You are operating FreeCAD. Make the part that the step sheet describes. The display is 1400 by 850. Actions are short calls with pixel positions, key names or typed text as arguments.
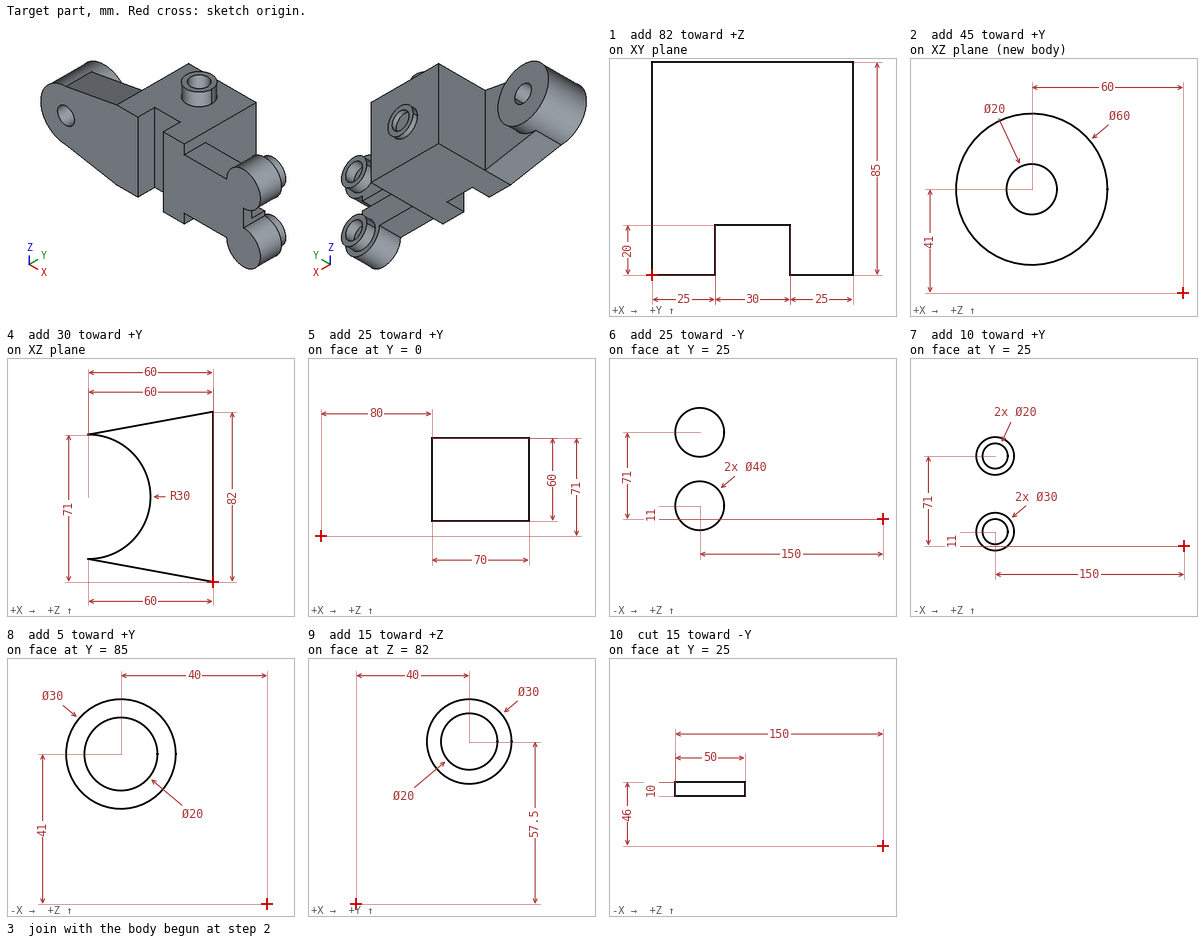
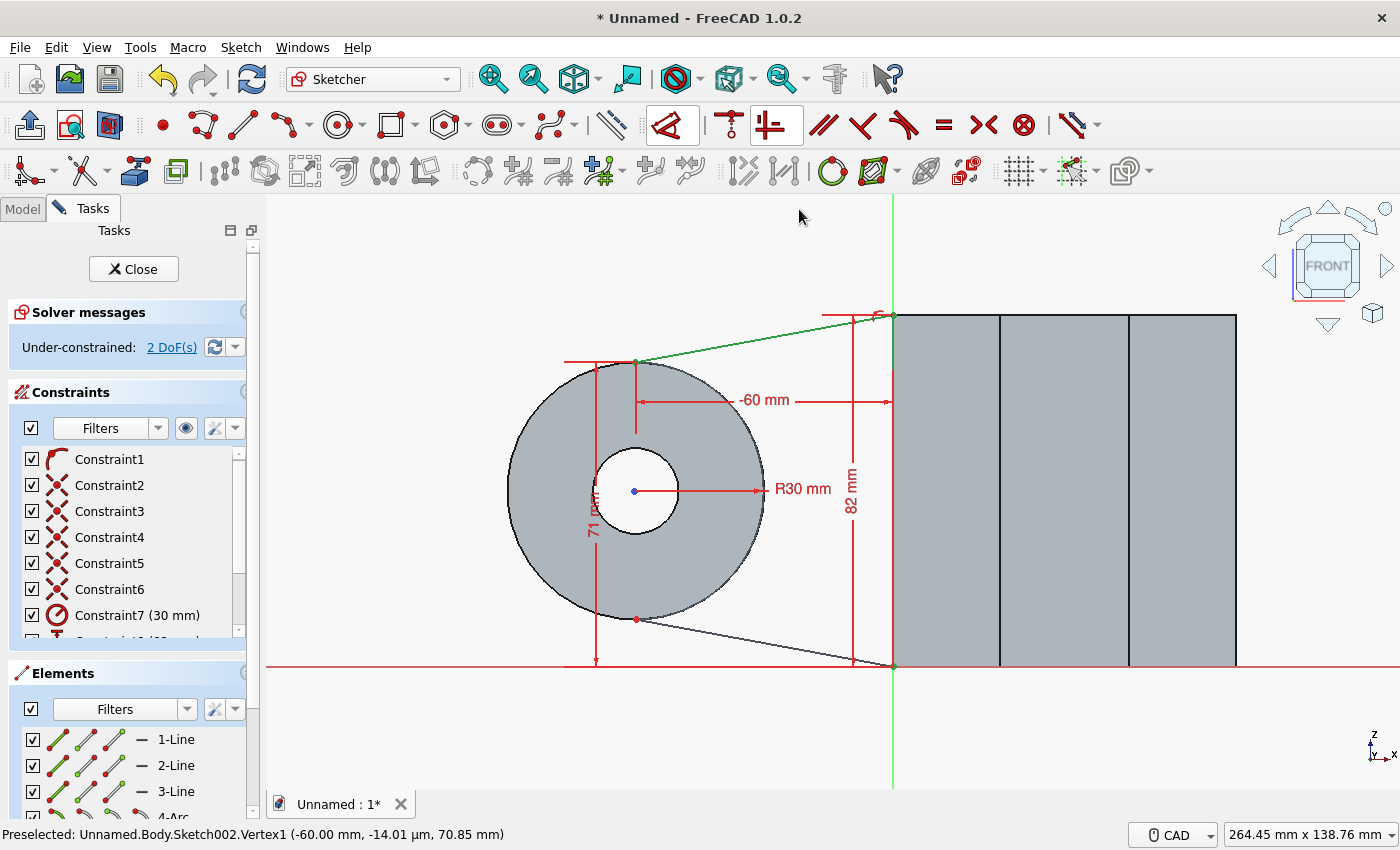
click(636, 620)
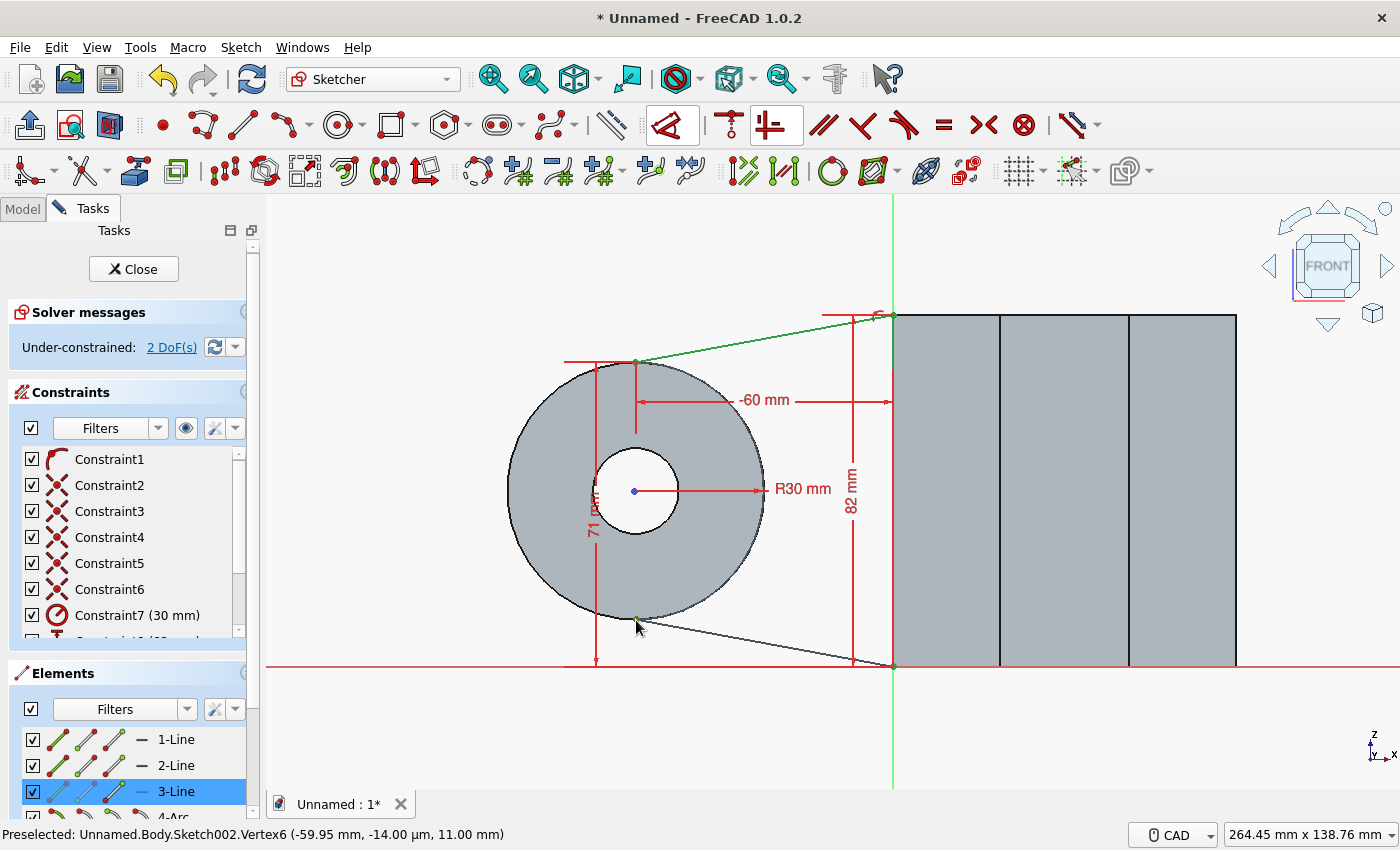
click(694, 126)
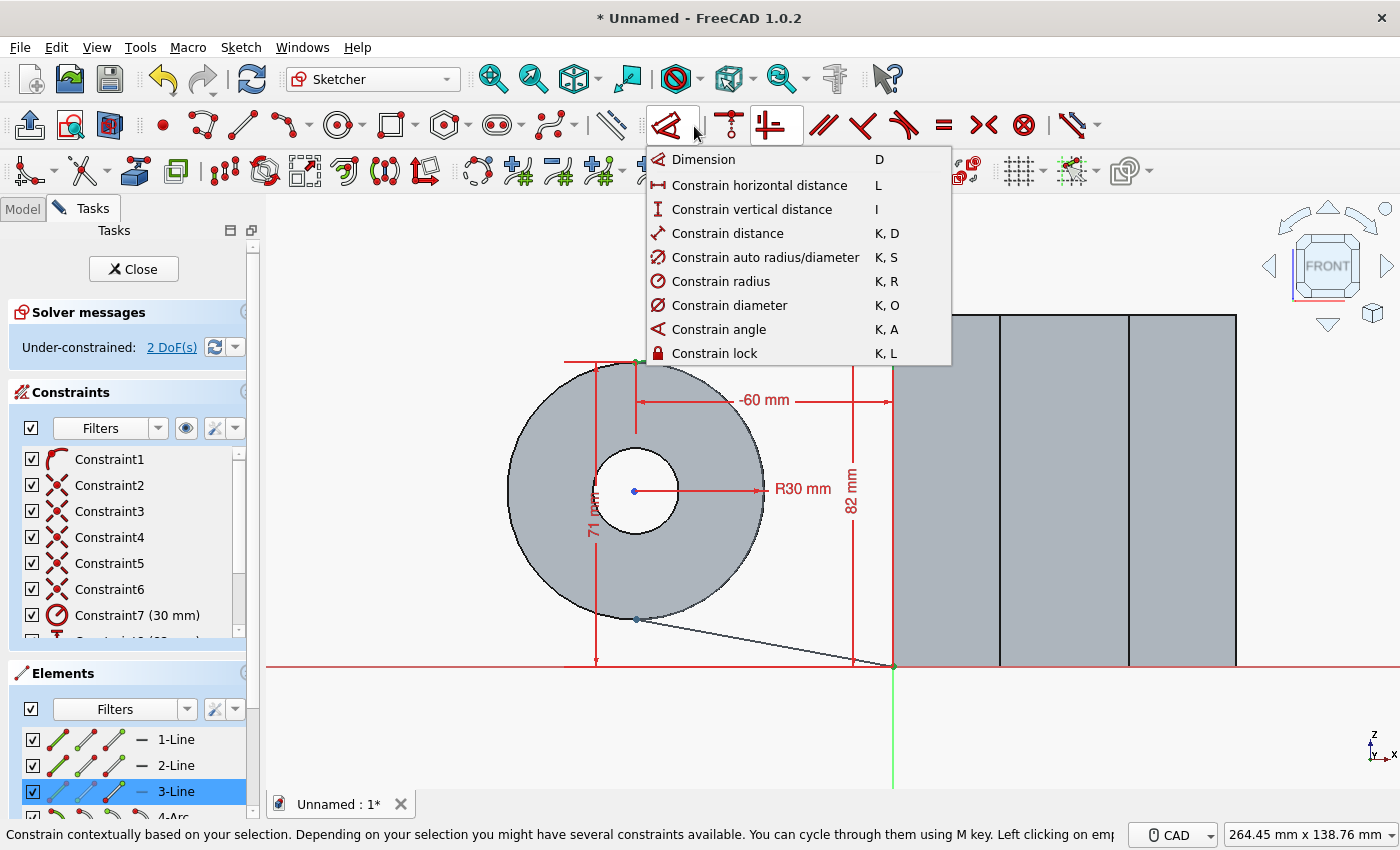
click(799, 185)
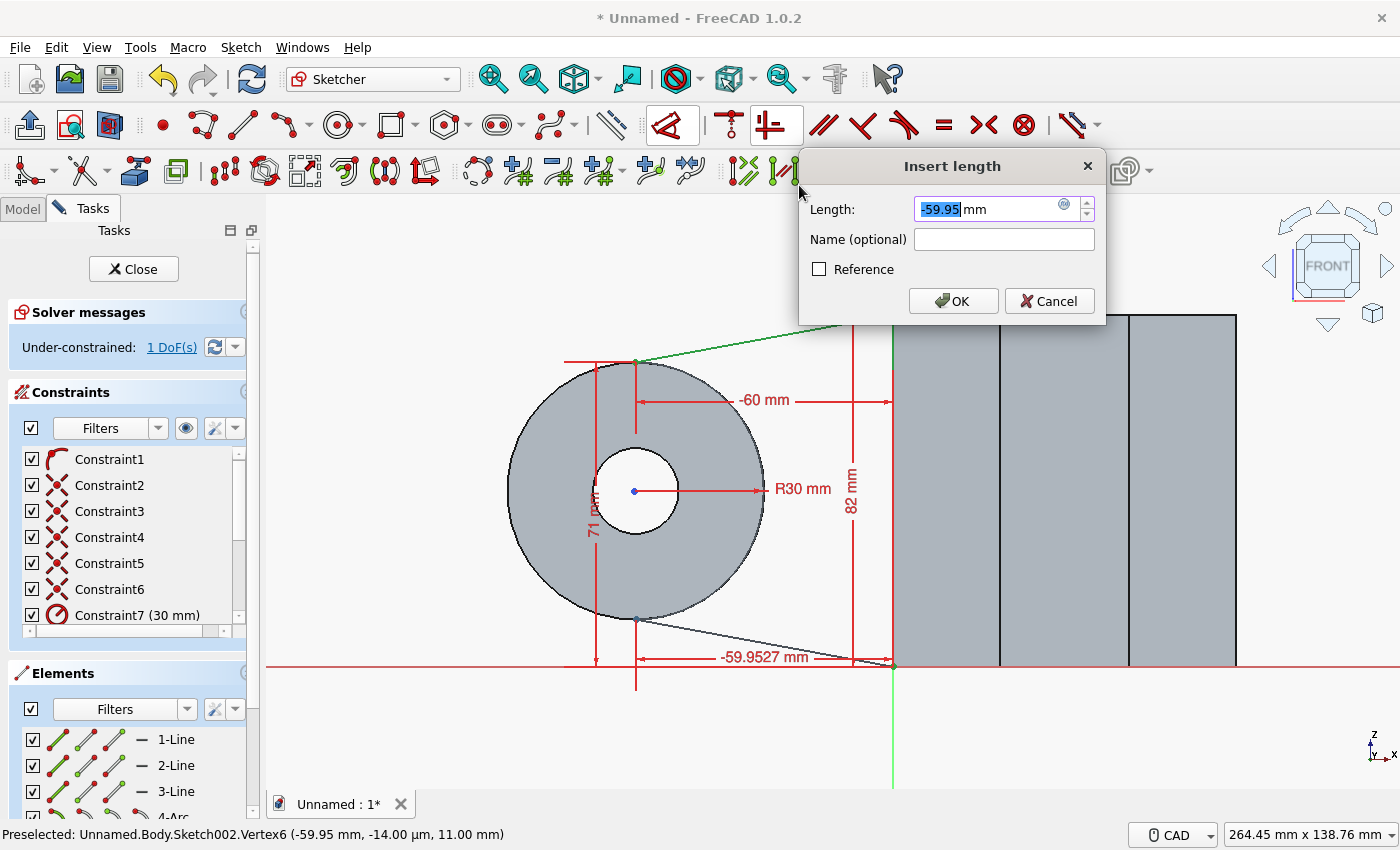
text(-60)
key(Return)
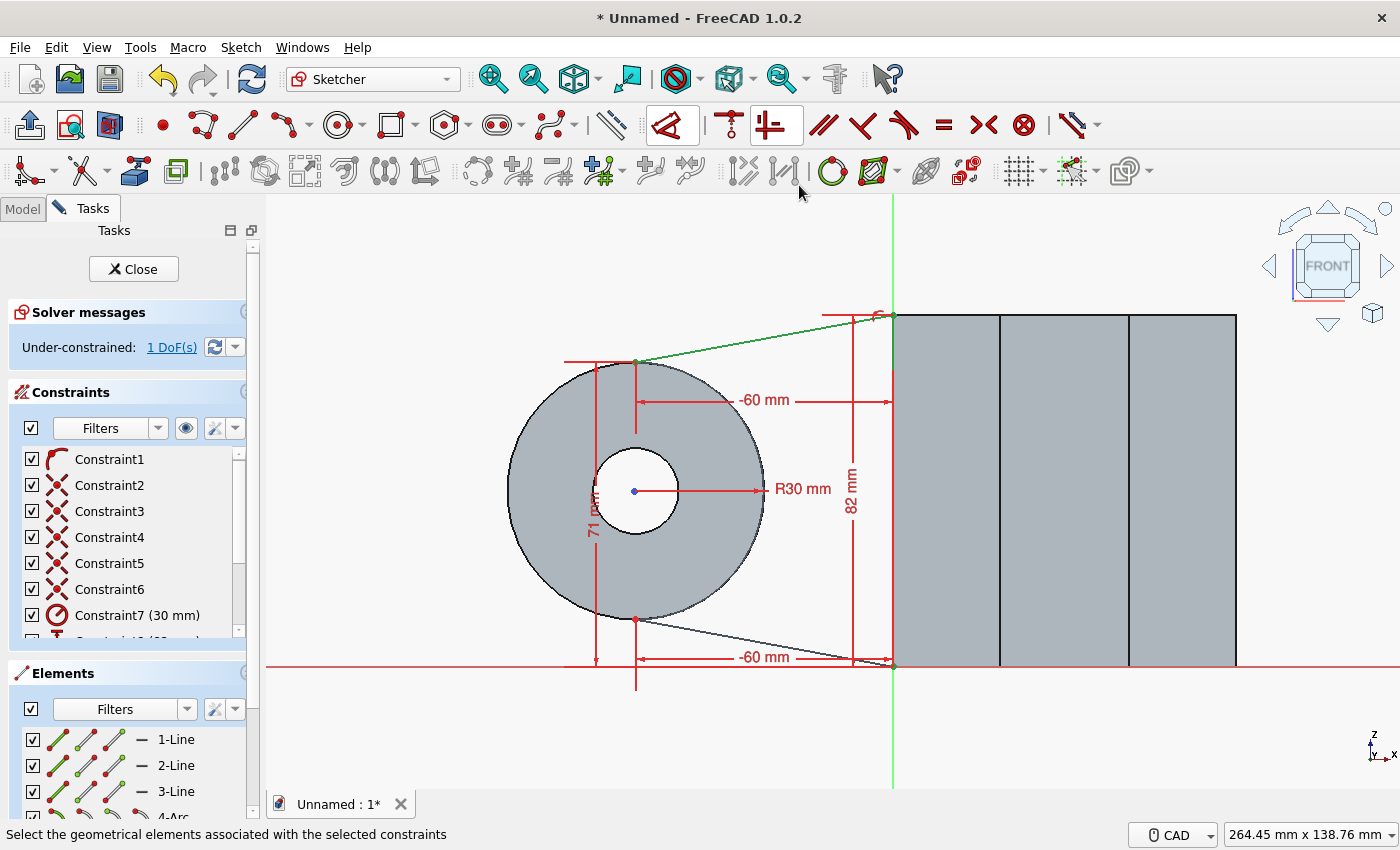
click(635, 491)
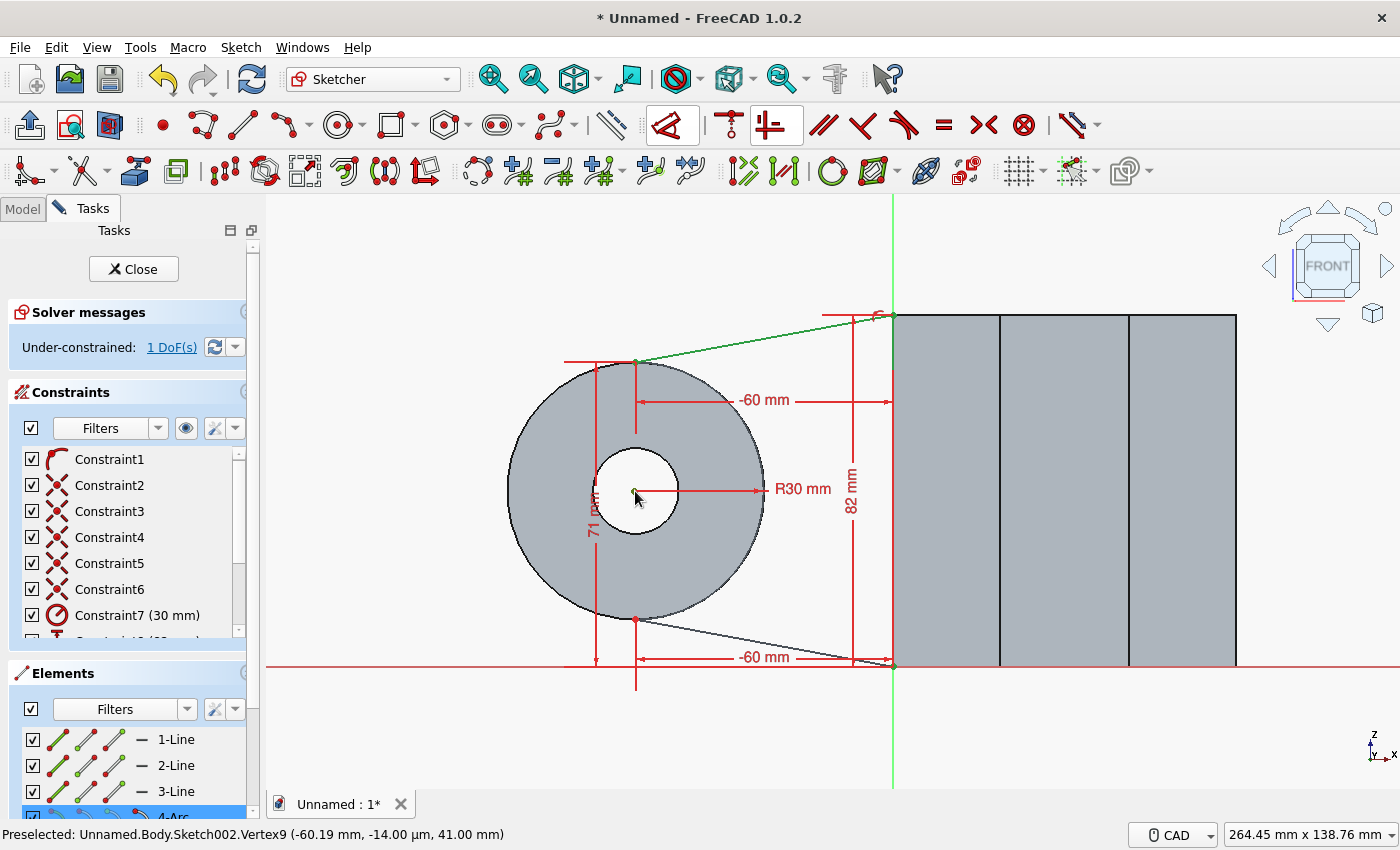
click(694, 126)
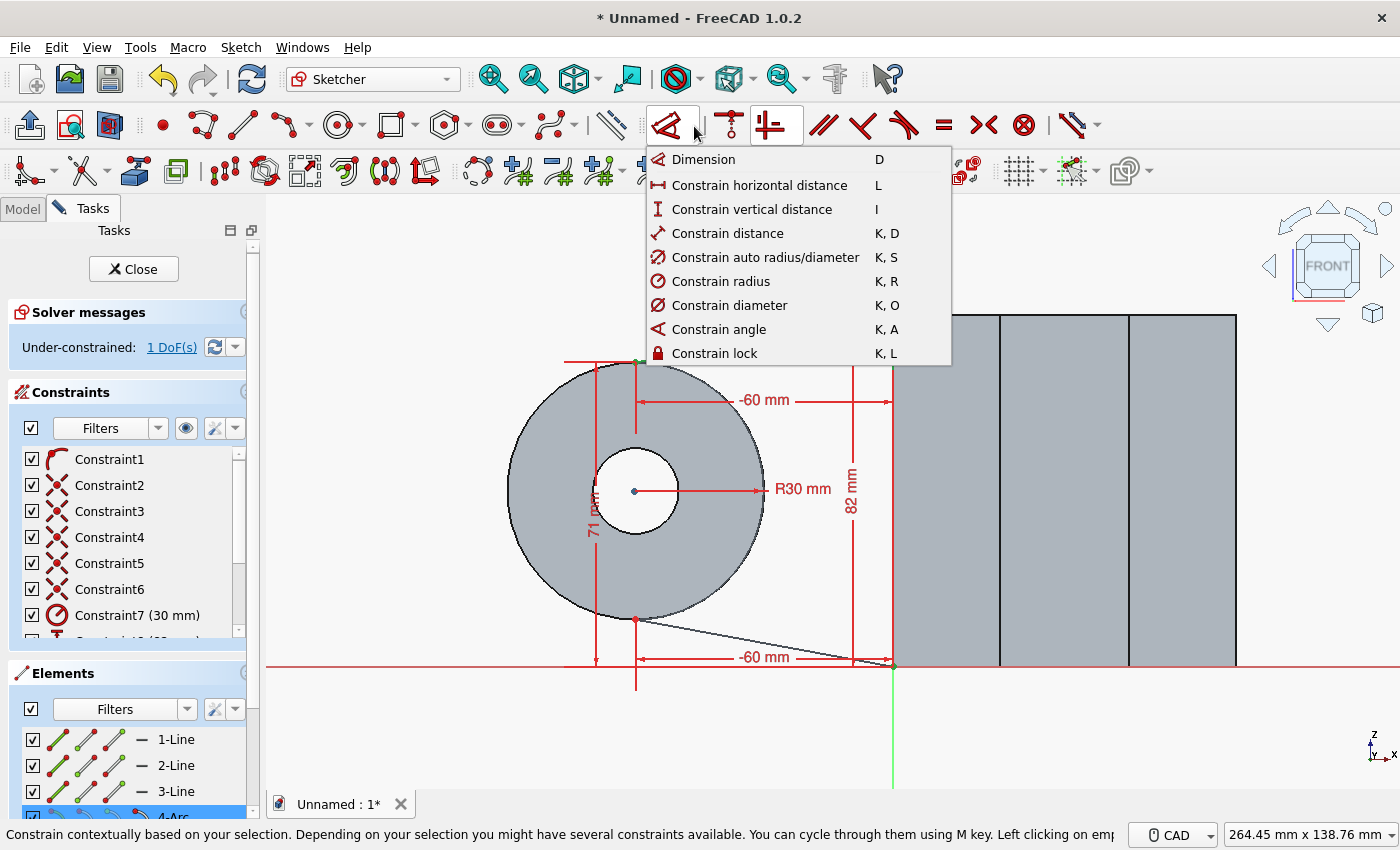
click(799, 185)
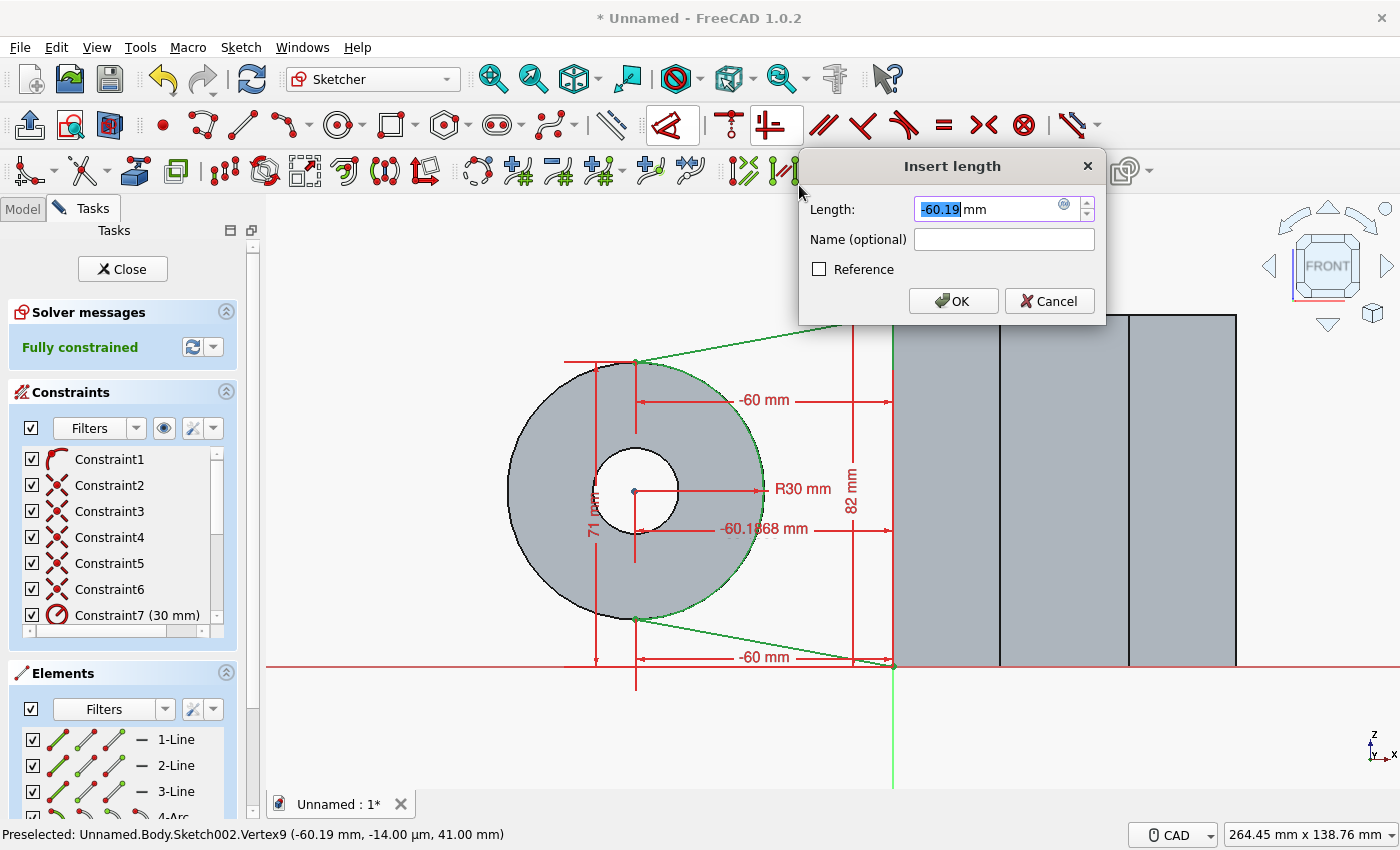
text(-60)
key(Return)